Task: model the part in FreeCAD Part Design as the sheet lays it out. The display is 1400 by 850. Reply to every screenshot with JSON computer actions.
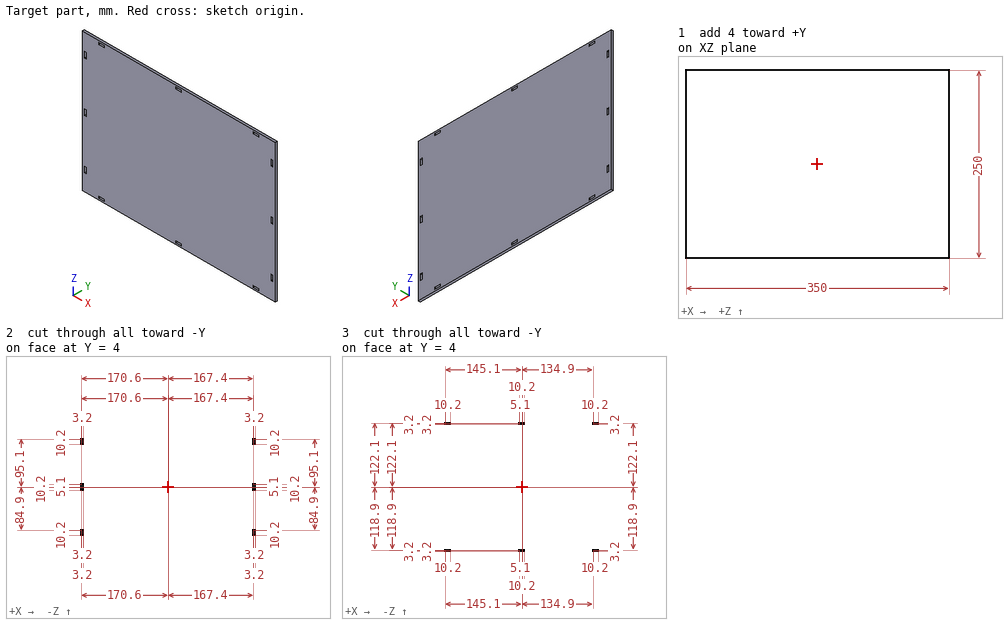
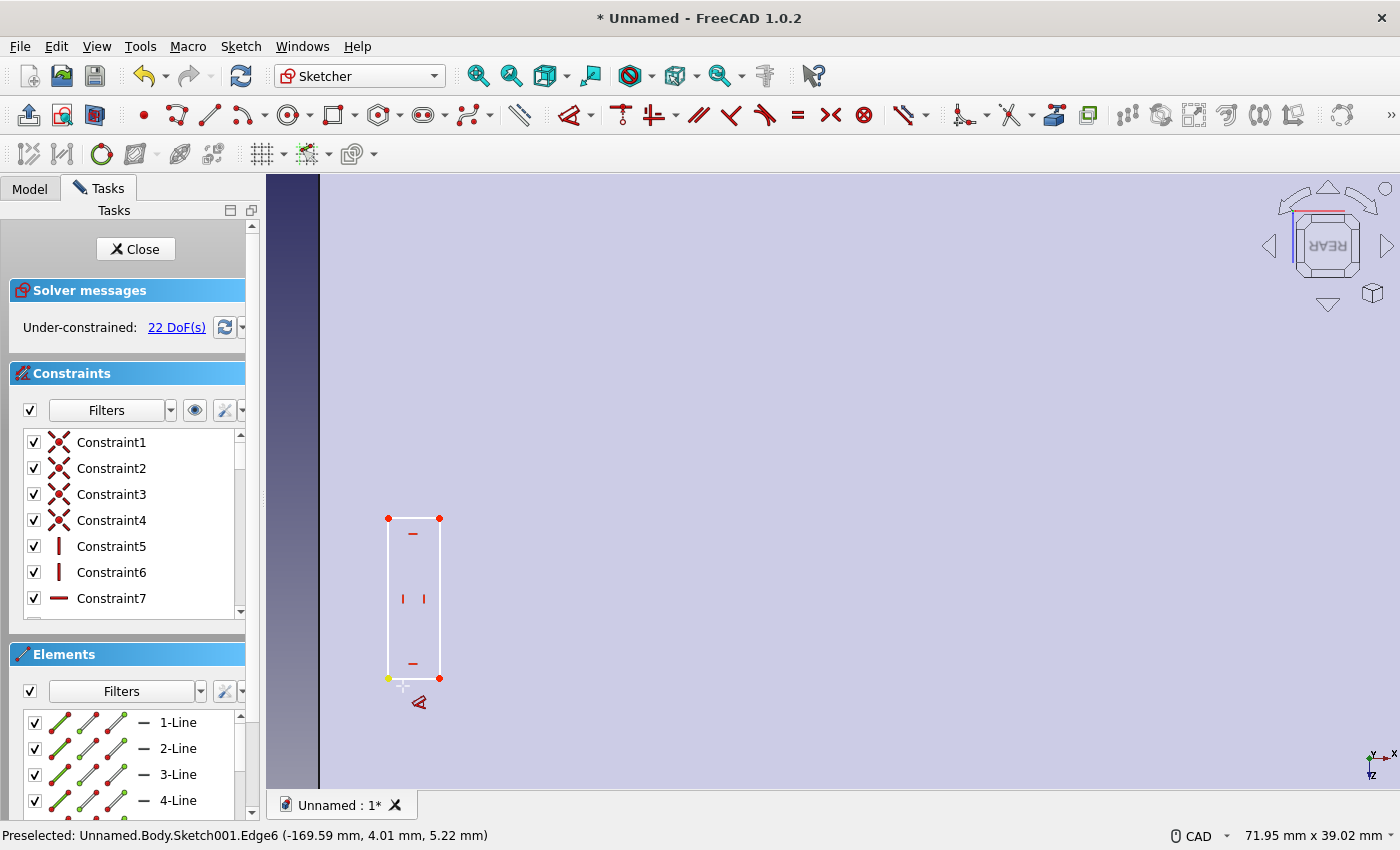
{"action": "left_click", "coordinate": [404, 679]}
{"action": "left_click", "coordinate": [414, 713]}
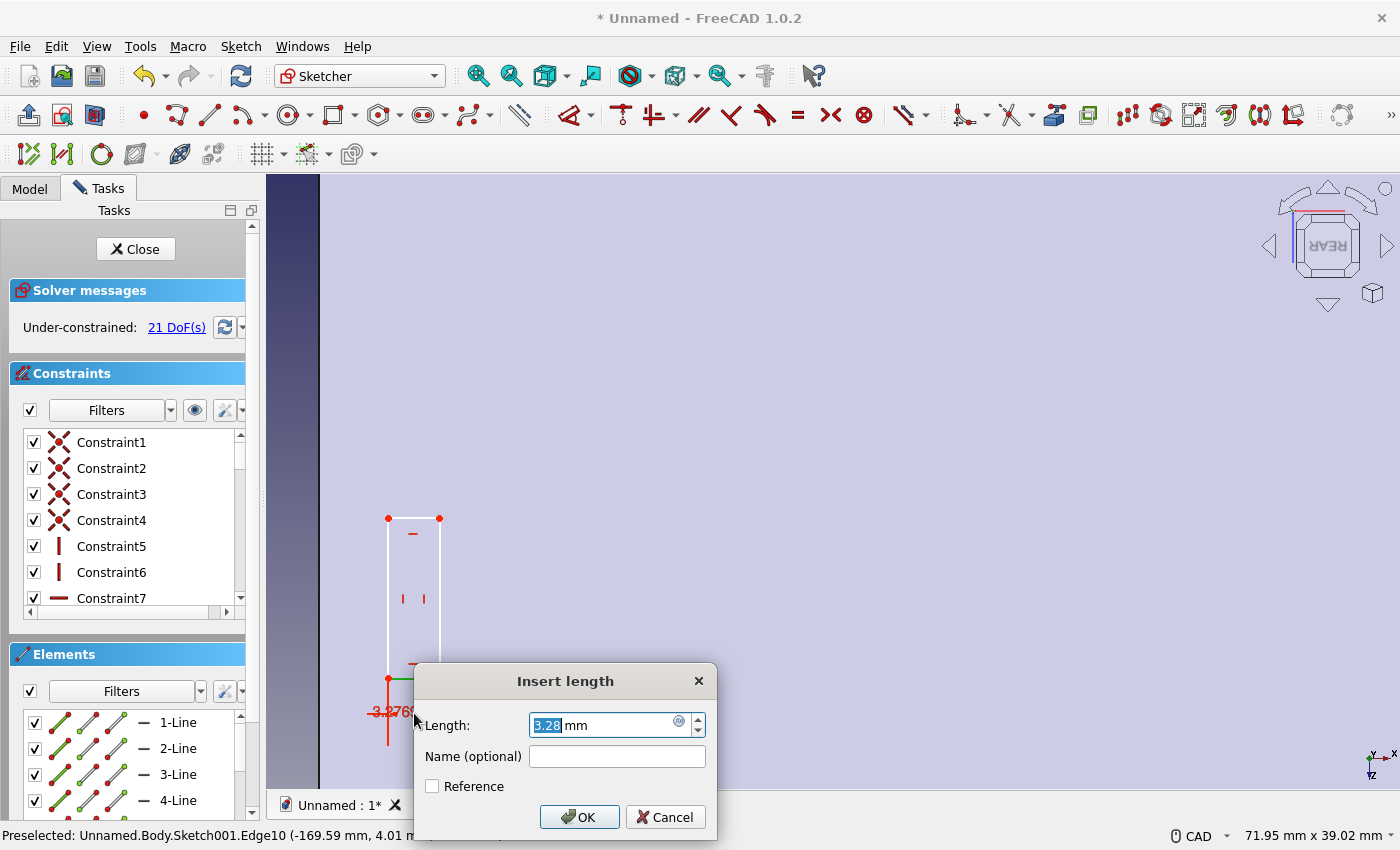
{"action": "type", "text": "3.2"}
{"action": "key", "text": "Return"}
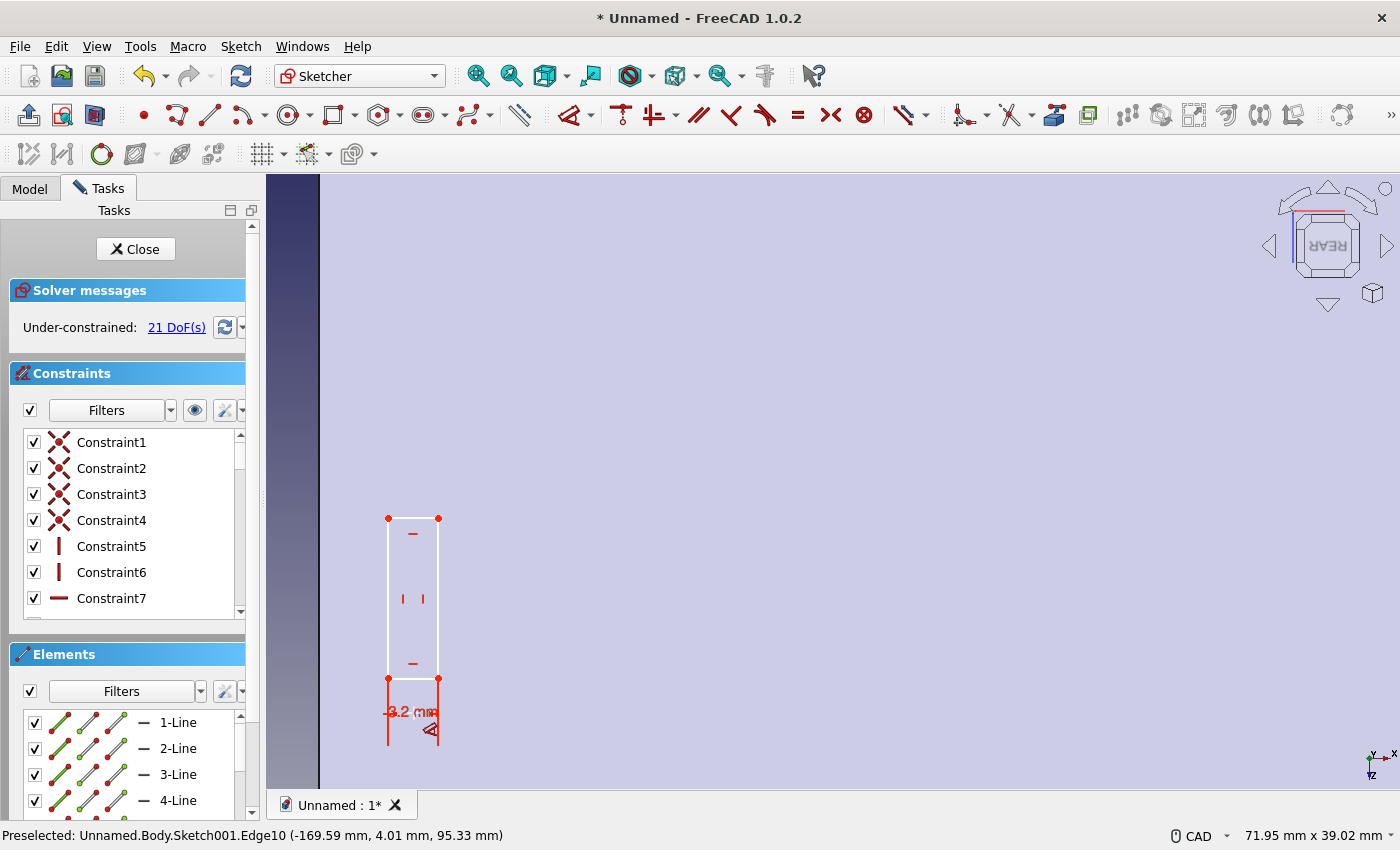
{"action": "scroll", "coordinate": [403, 686], "scroll_direction": "down", "scroll_amount": 10}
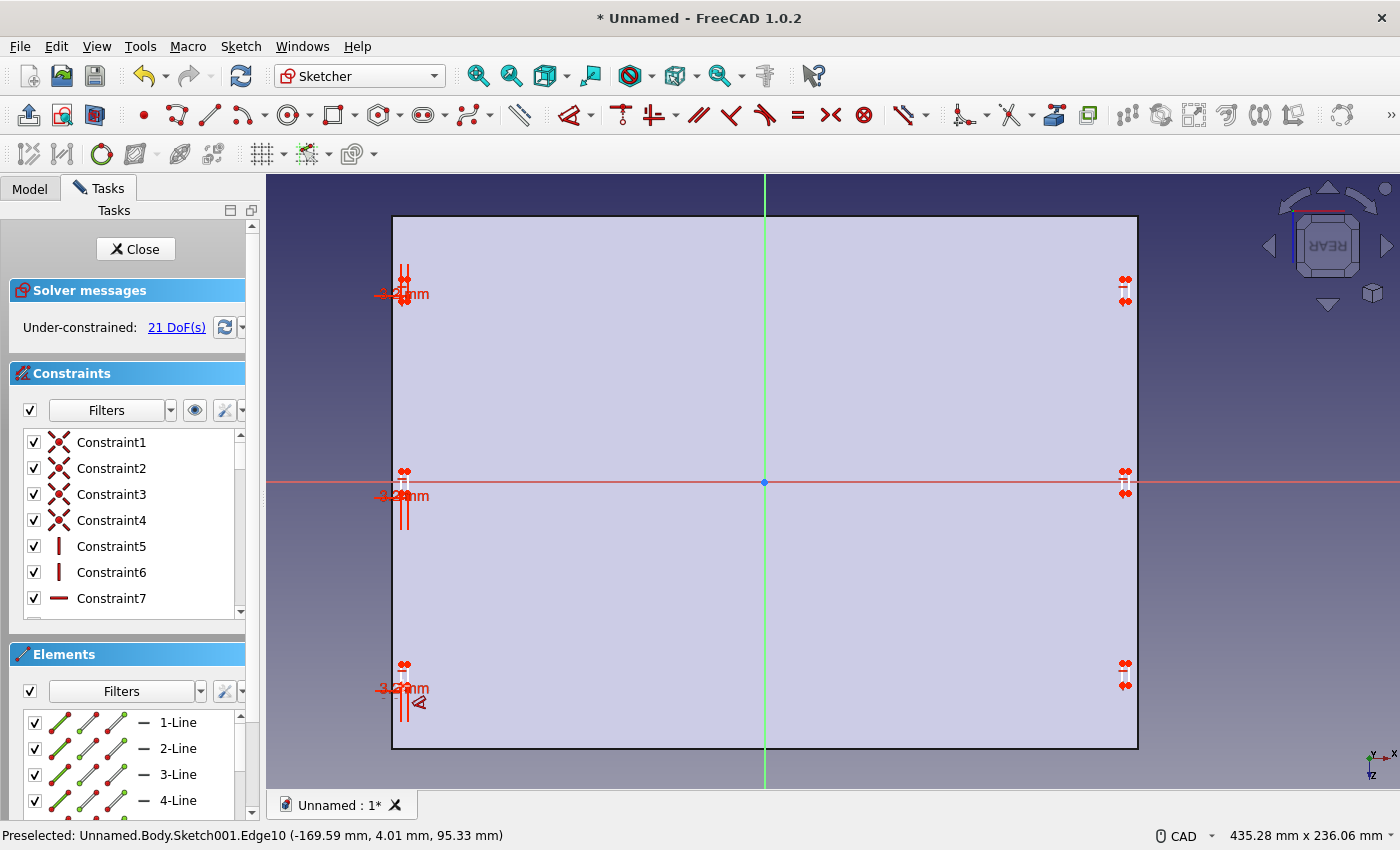
{"action": "scroll", "coordinate": [1124, 685], "scroll_direction": "up", "scroll_amount": 10}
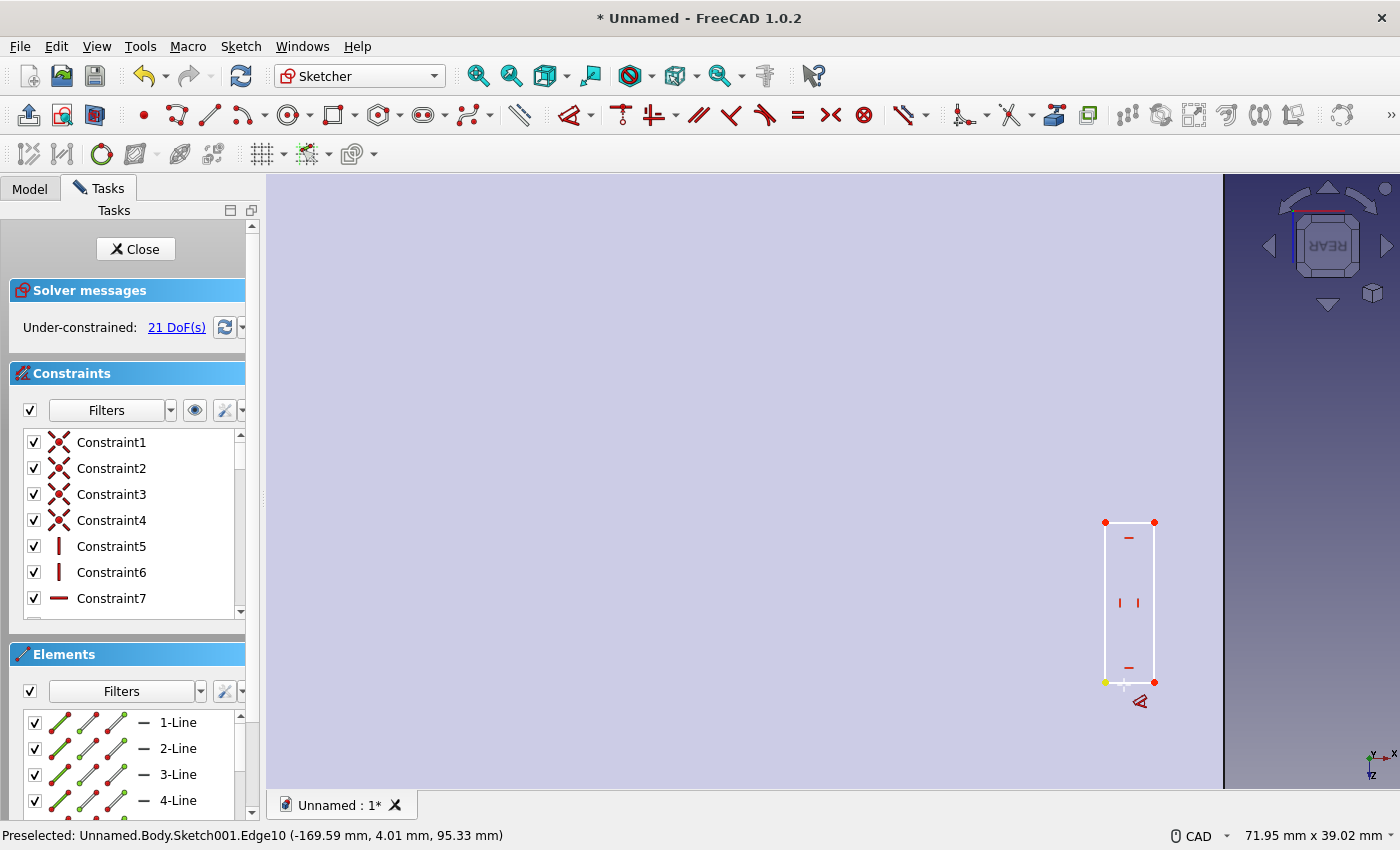
{"action": "left_click", "coordinate": [1120, 683]}
{"action": "left_click", "coordinate": [1130, 717]}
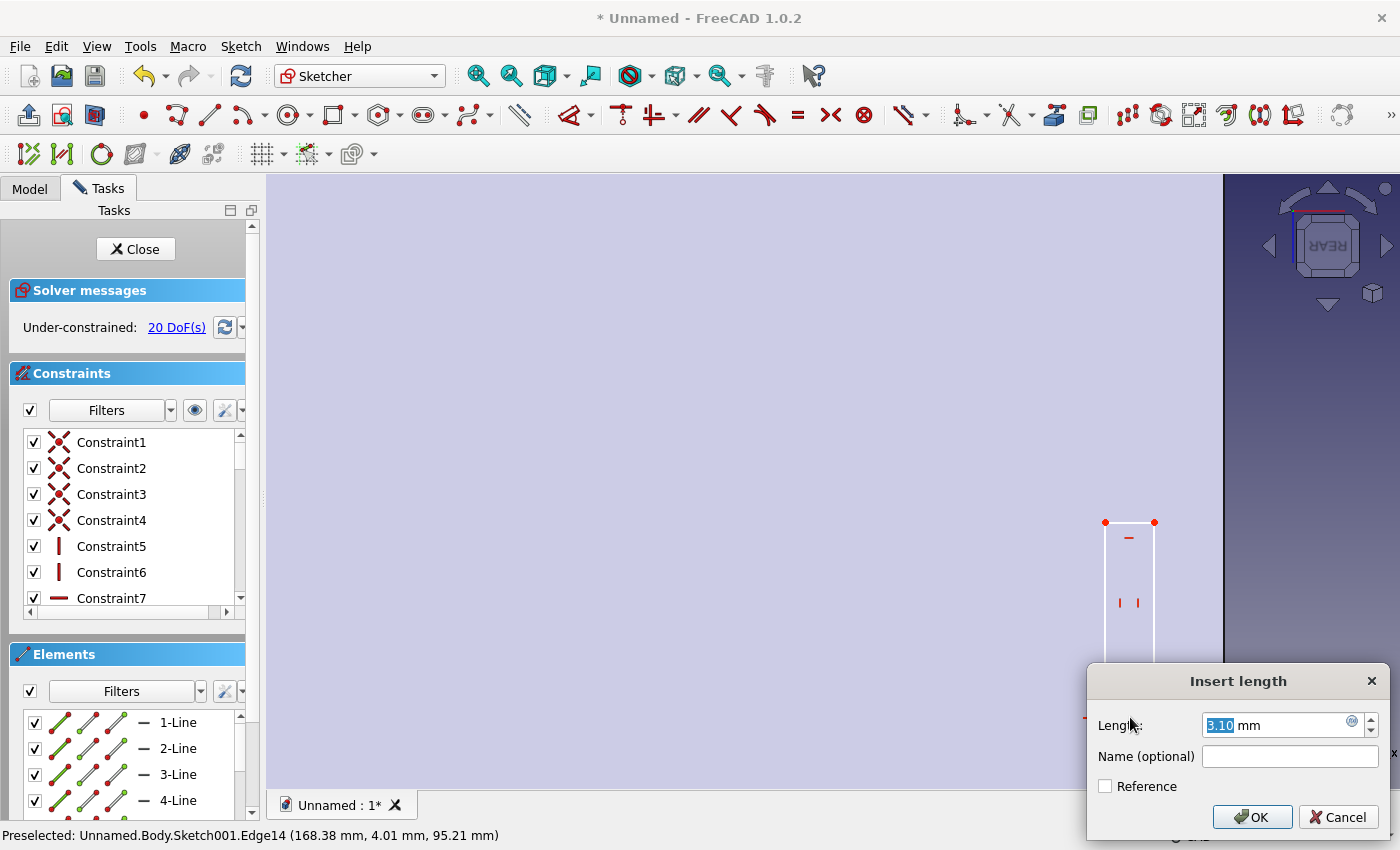
{"action": "type", "text": "3.2"}
{"action": "key", "text": "Return"}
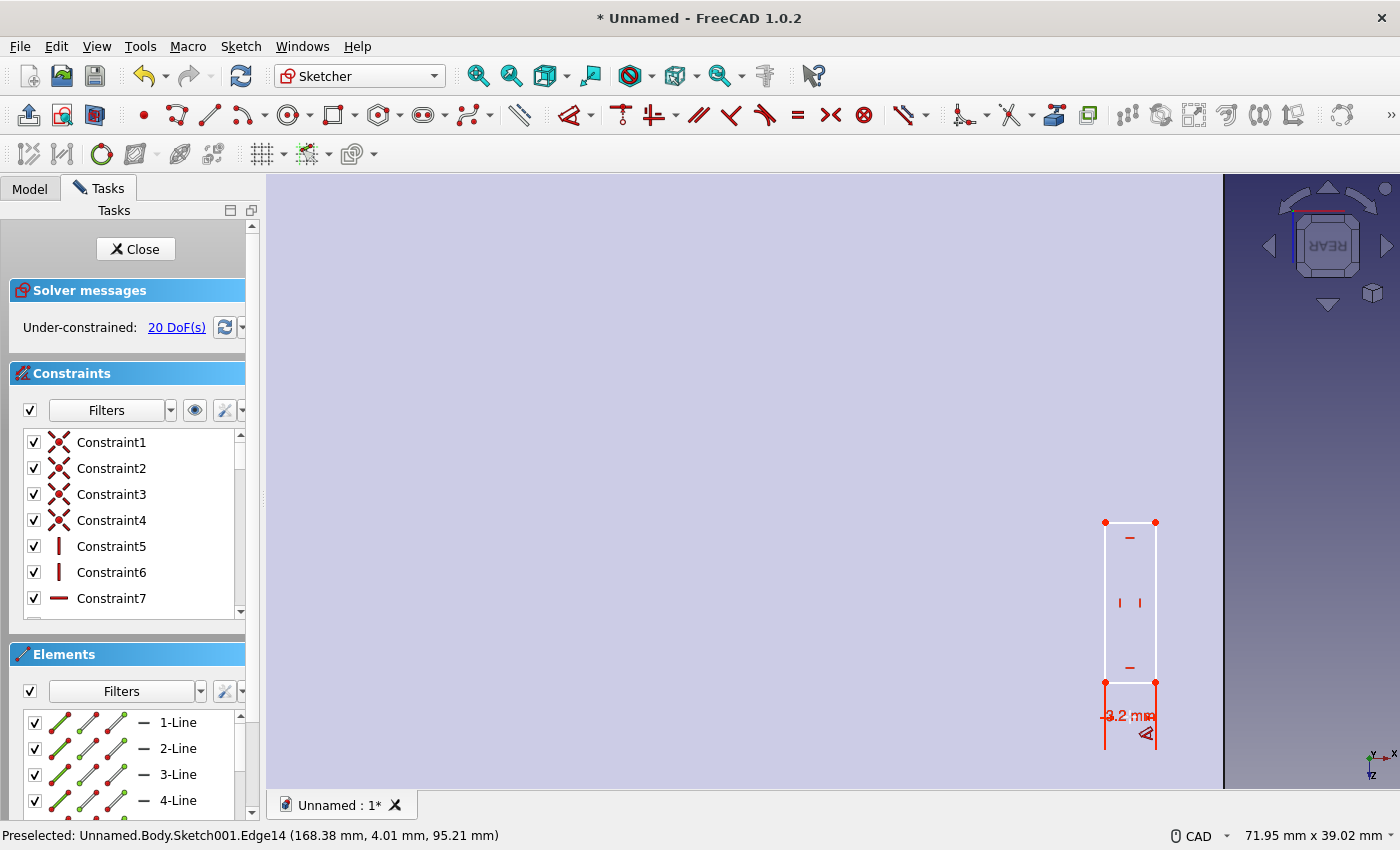
{"action": "scroll", "coordinate": [1124, 685], "scroll_direction": "down", "scroll_amount": 10}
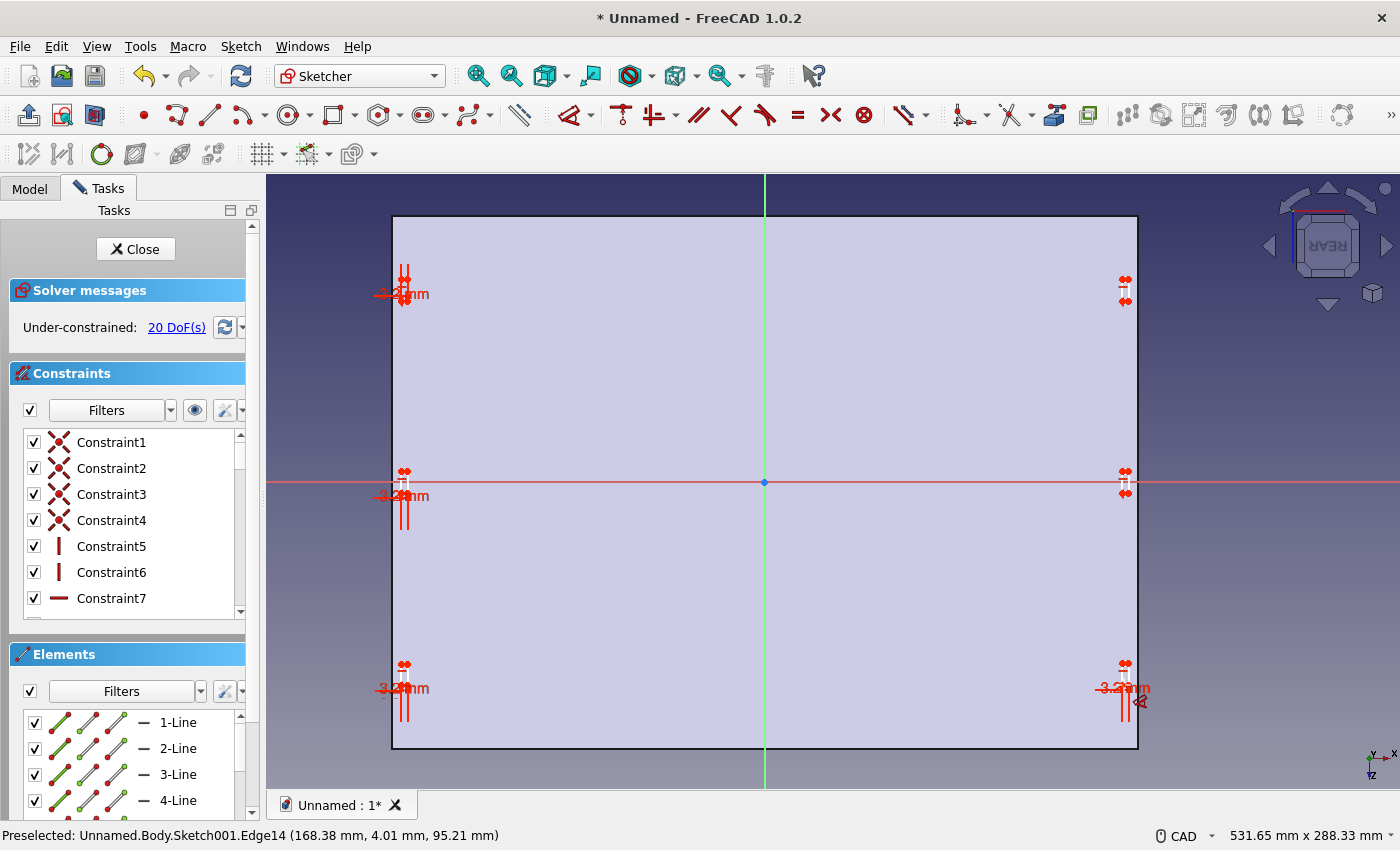
{"action": "scroll", "coordinate": [1124, 494], "scroll_direction": "up", "scroll_amount": 10}